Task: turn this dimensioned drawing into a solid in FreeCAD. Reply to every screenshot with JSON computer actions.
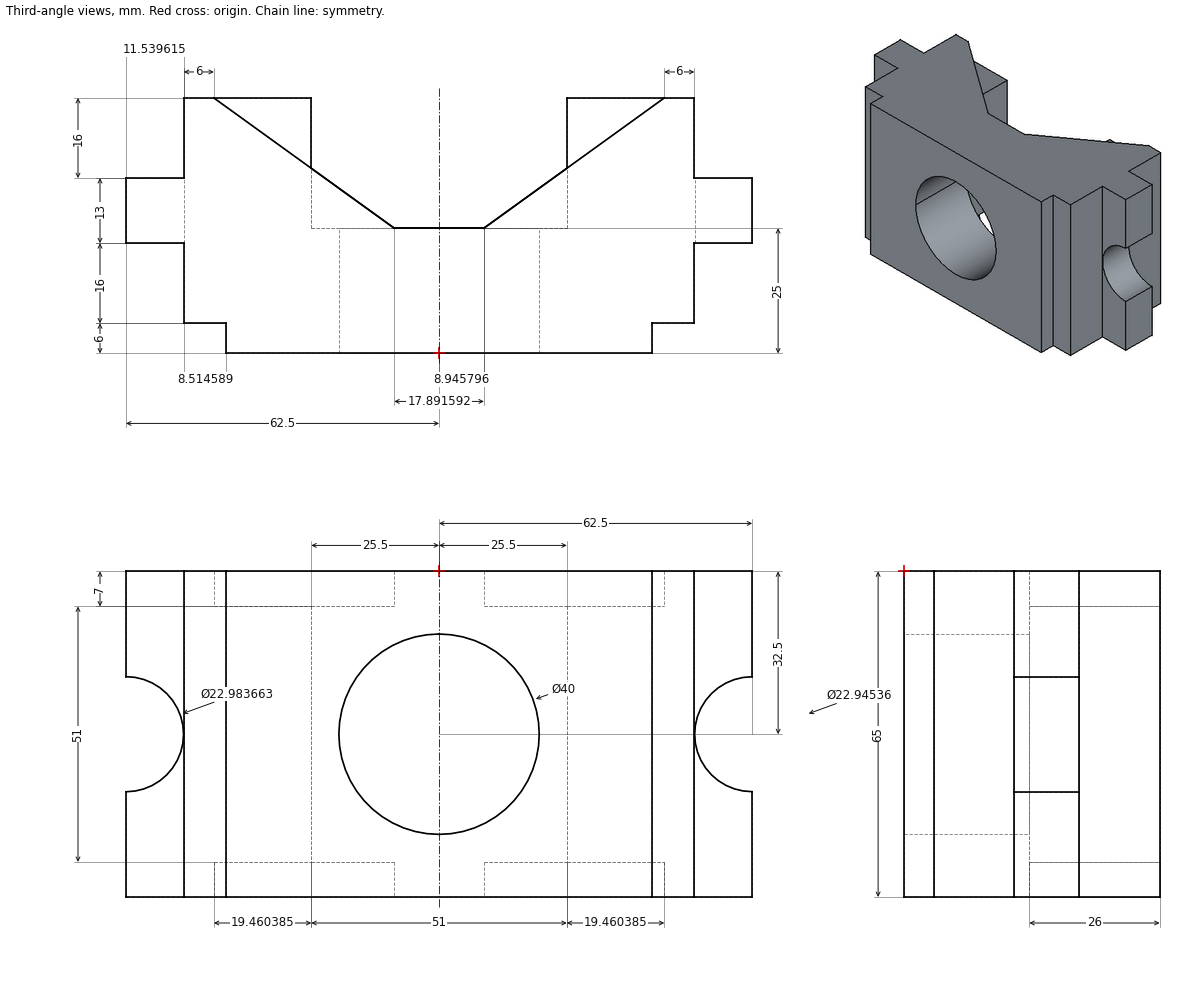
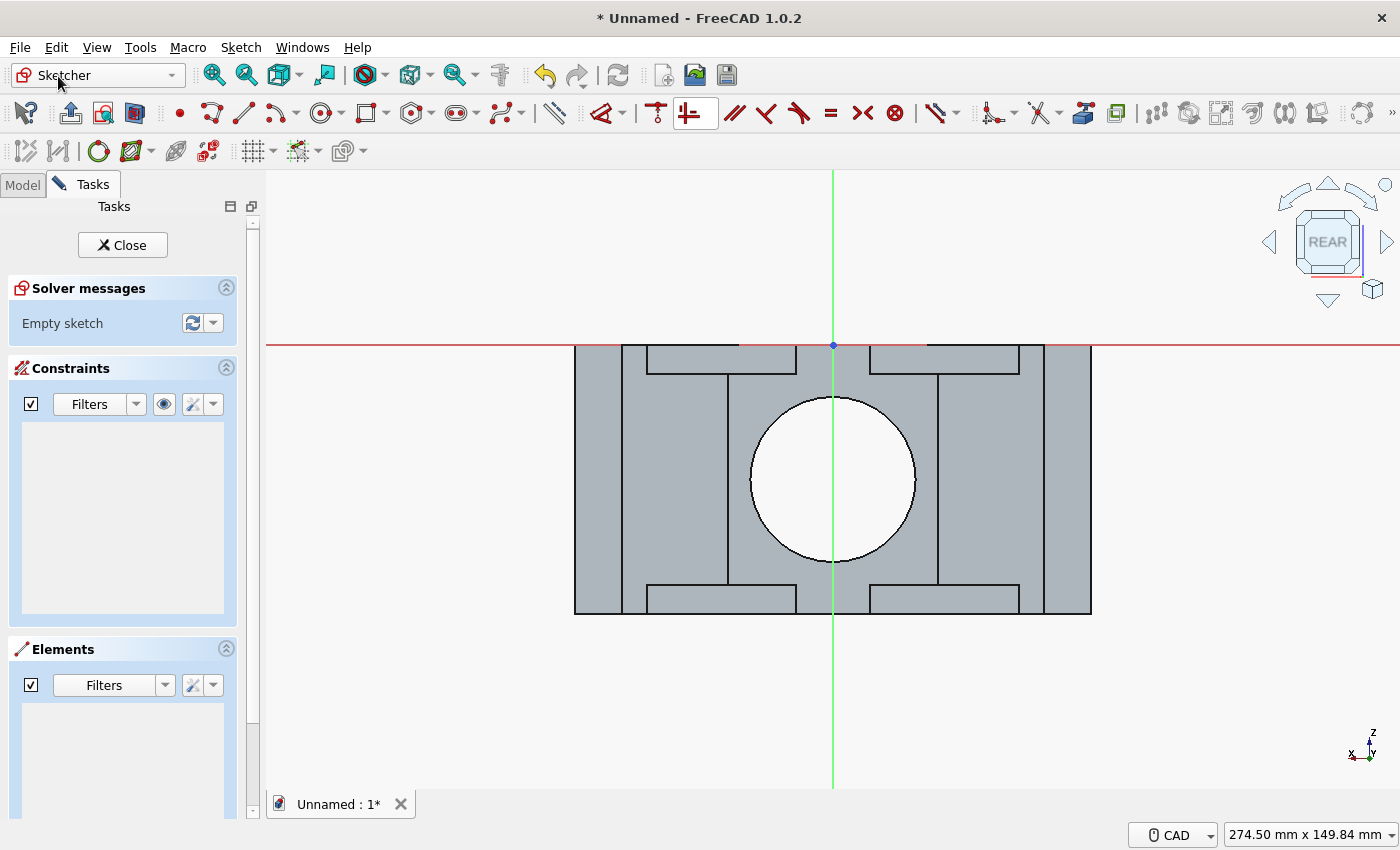
{"action": "left_click", "coordinate": [136, 114]}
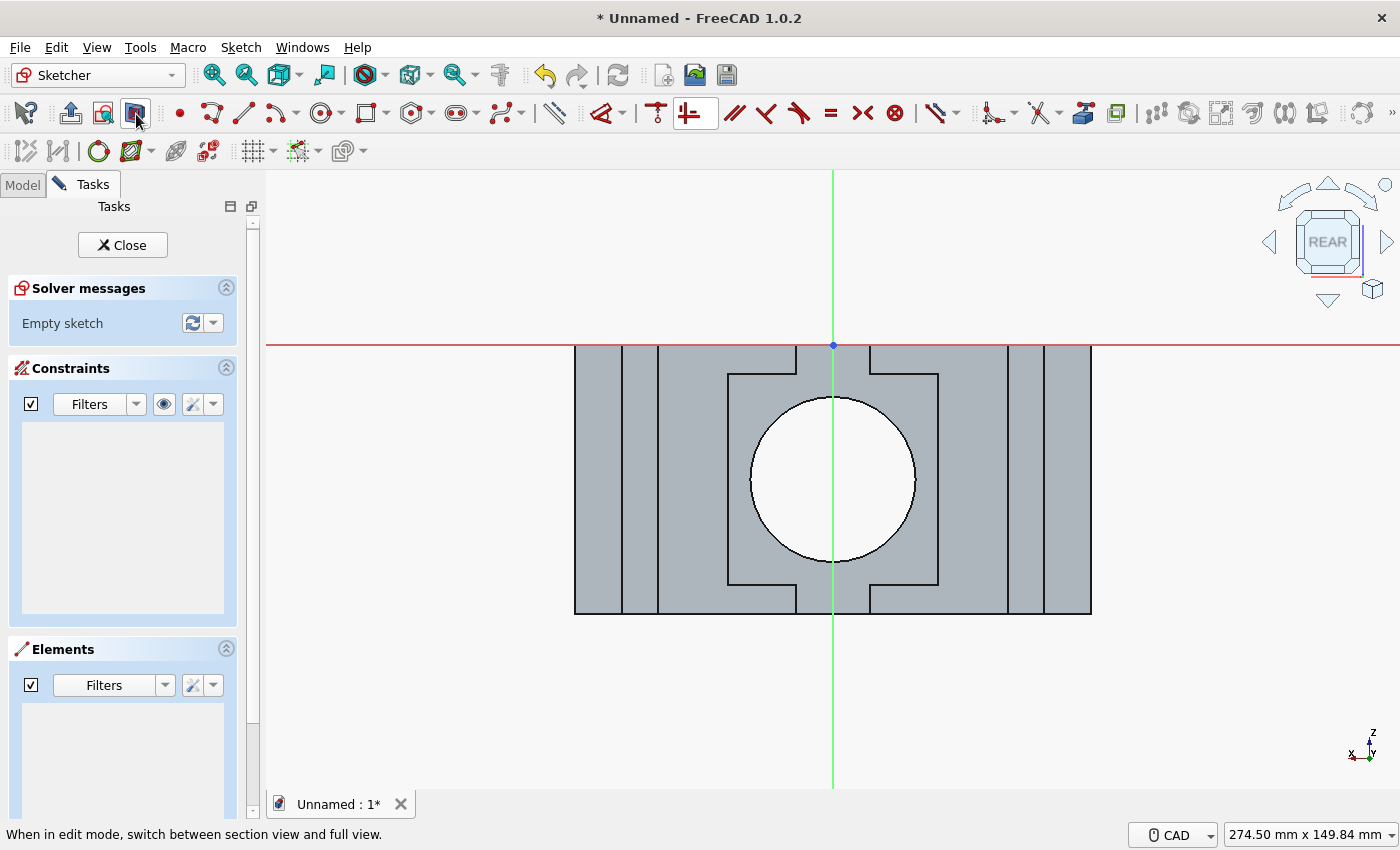
{"action": "left_click", "coordinate": [322, 114]}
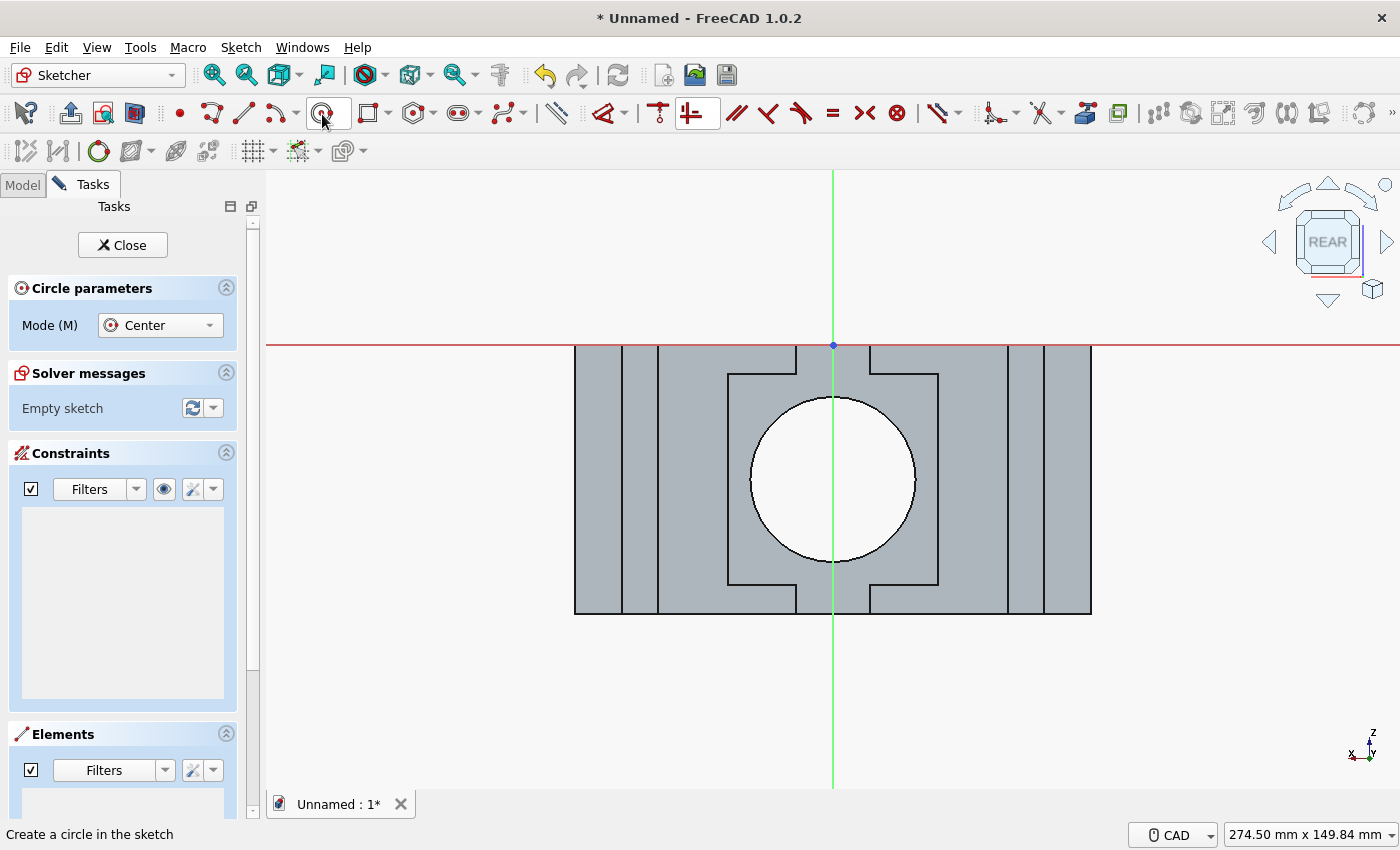
{"action": "left_click", "coordinate": [575, 480]}
{"action": "mouse_move", "coordinate": [608, 446]}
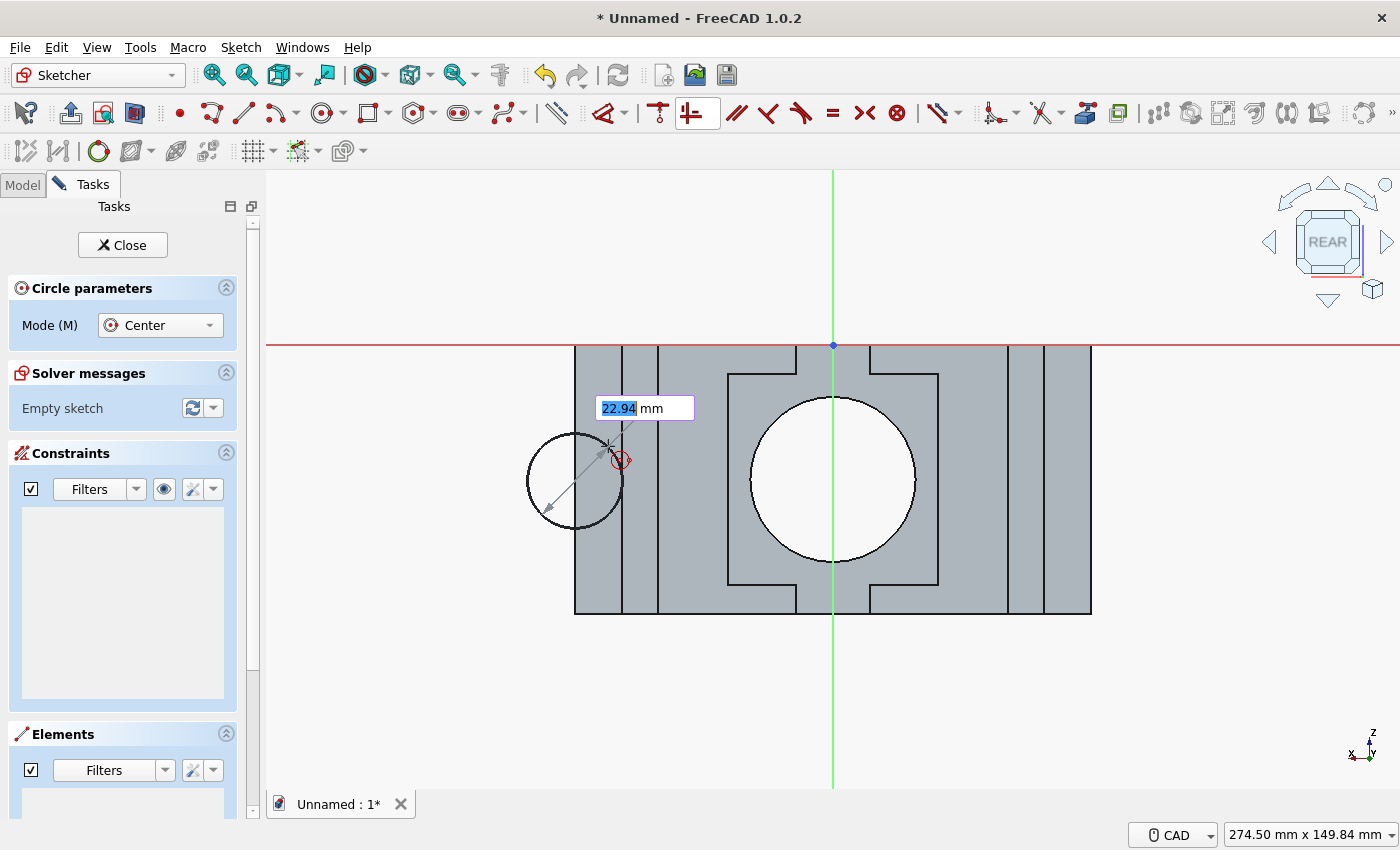
{"action": "type", "text": "22.94536"}
{"action": "key", "text": "Return"}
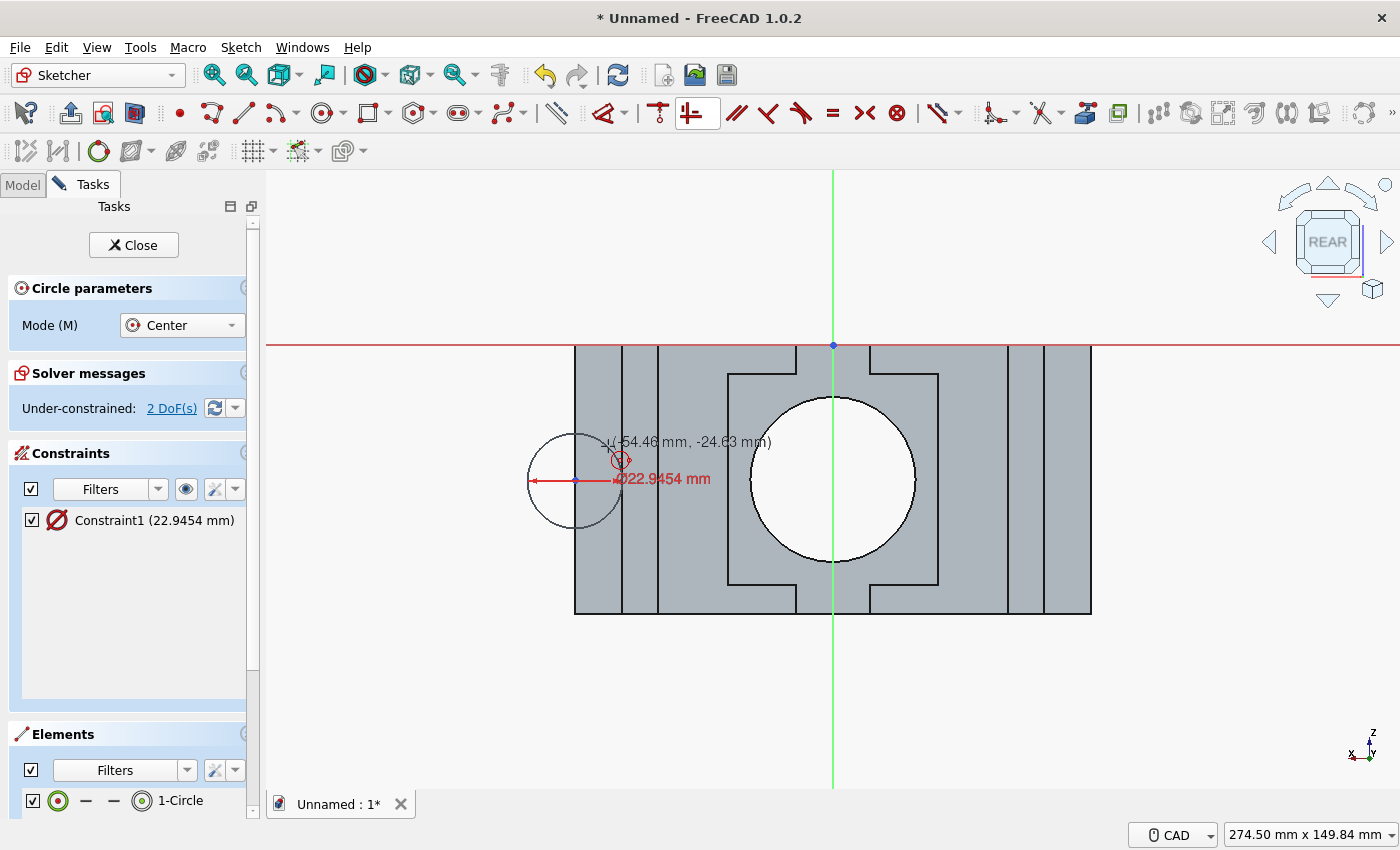
{"action": "left_click", "coordinate": [1091, 480]}
{"action": "mouse_move", "coordinate": [1125, 446]}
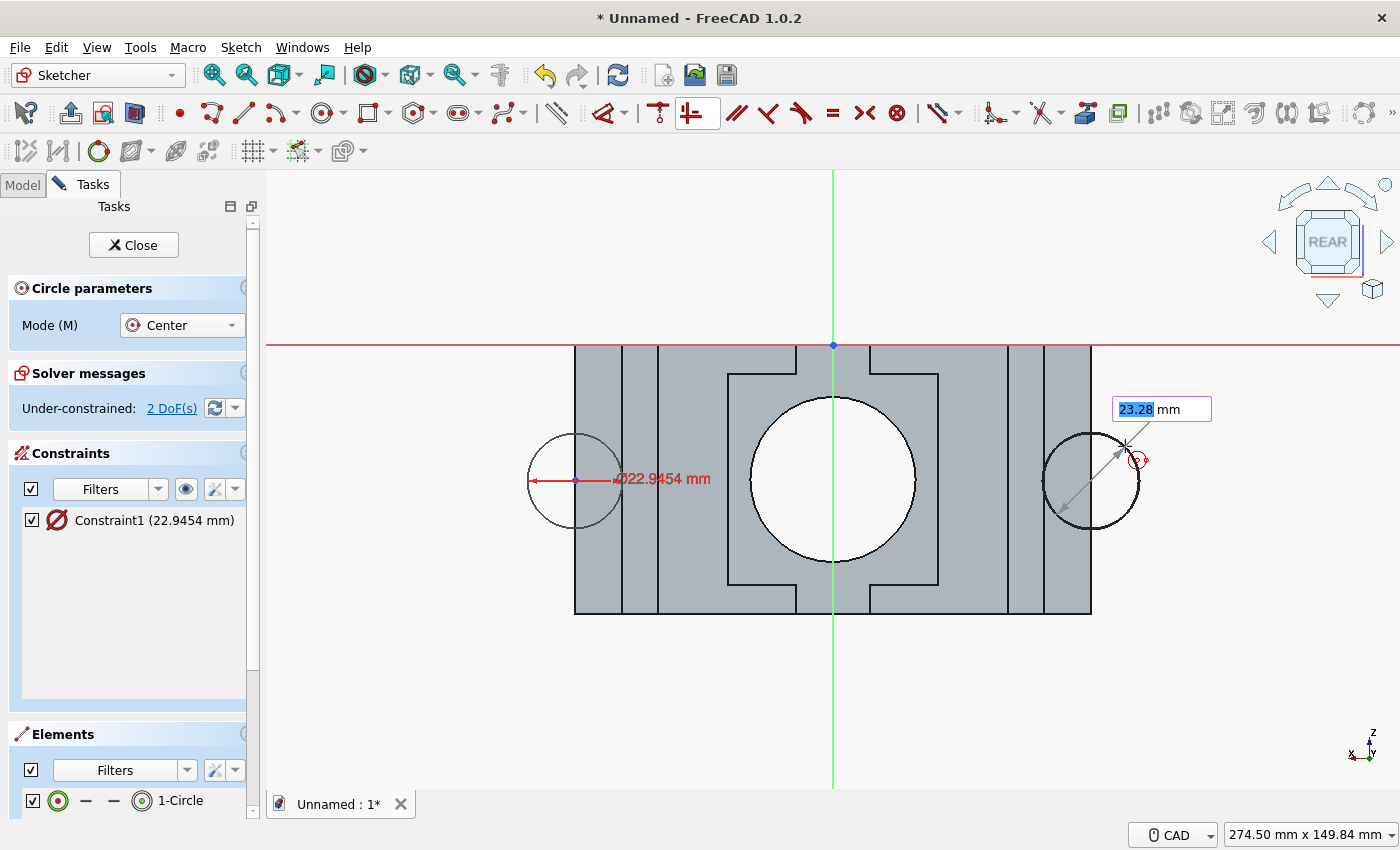
{"action": "type", "text": "22.983663"}
{"action": "key", "text": "Return"}
{"action": "key", "text": "Escape"}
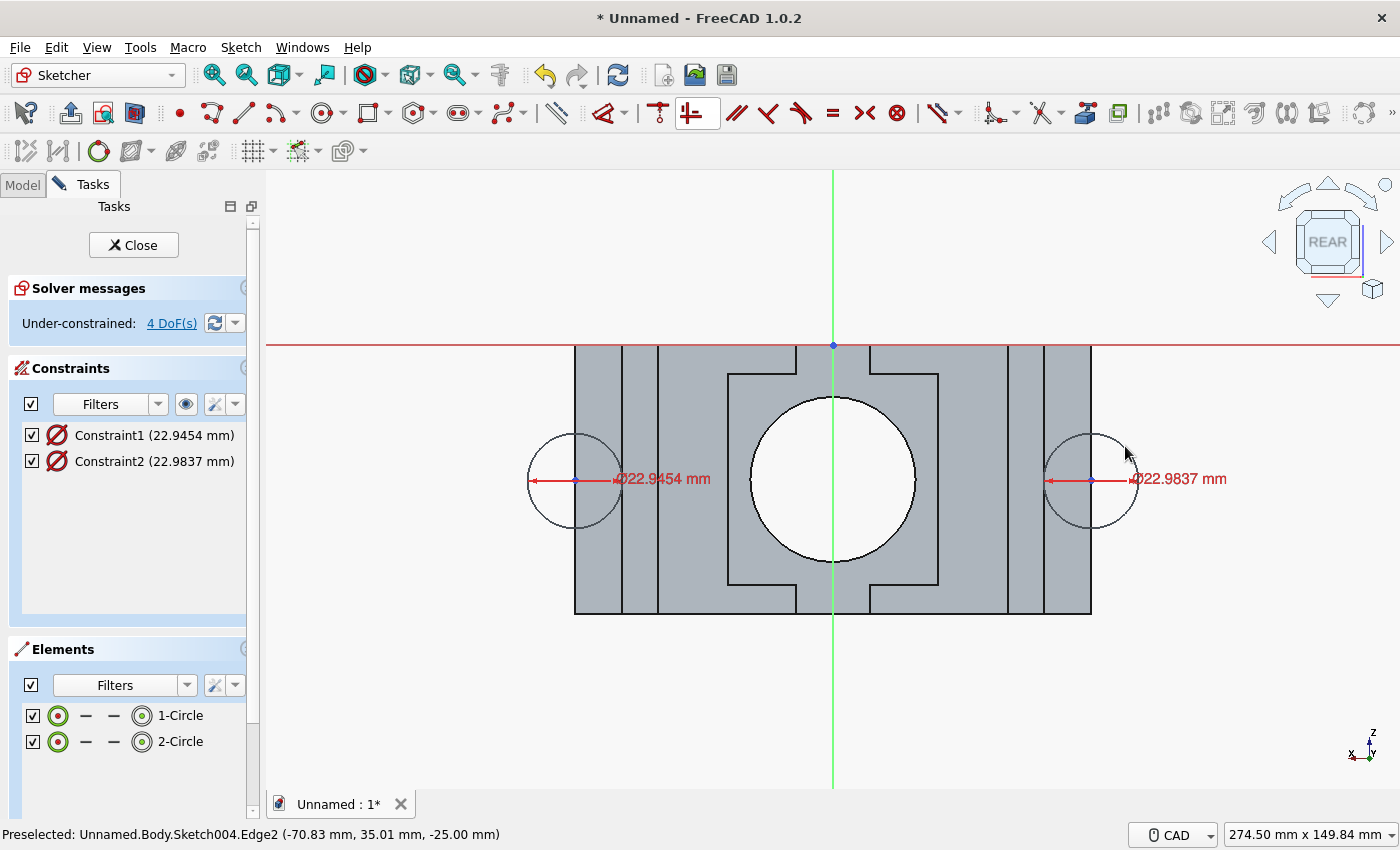
{"action": "left_click", "coordinate": [575, 481]}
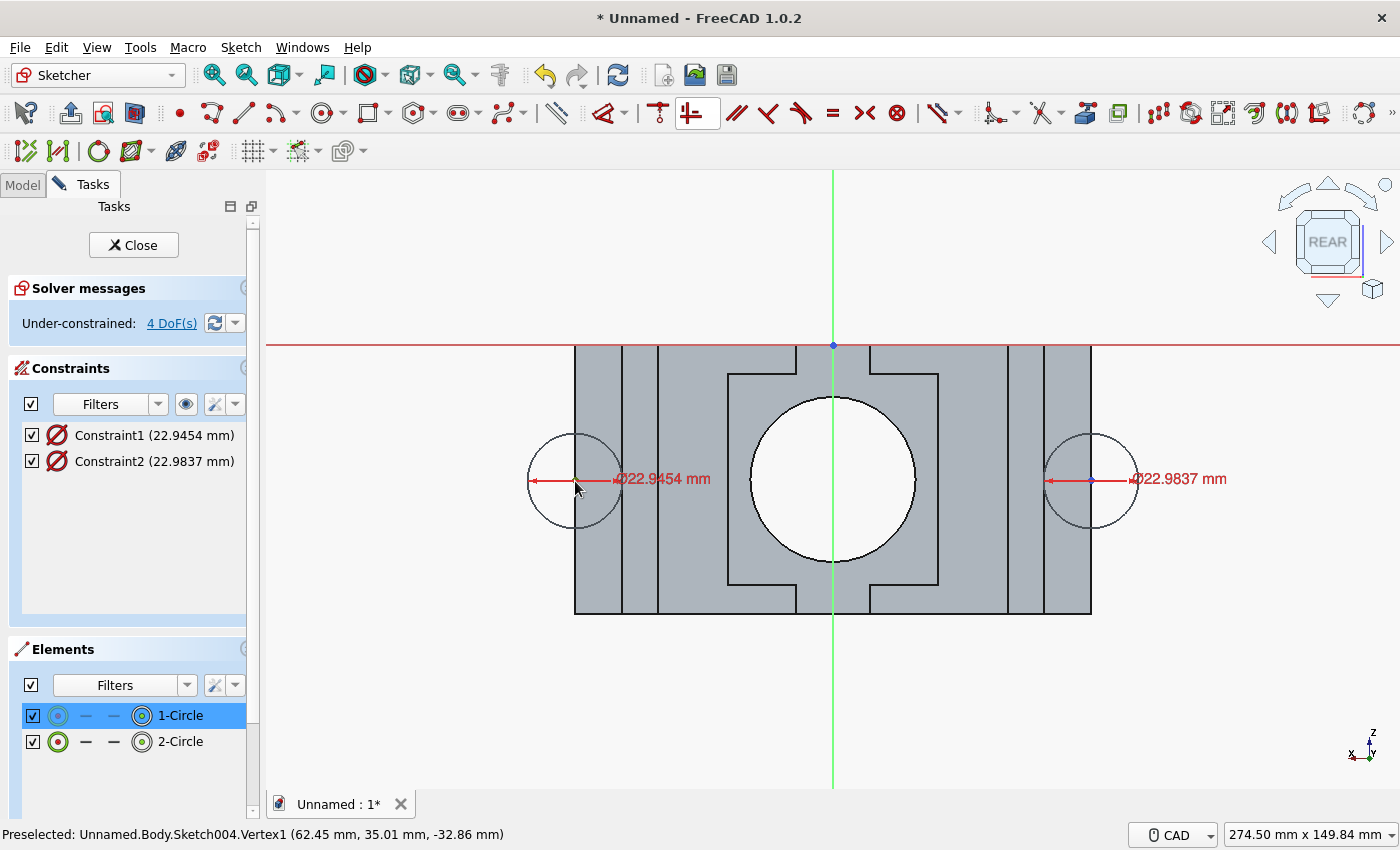
{"action": "left_click", "coordinate": [1091, 481]}